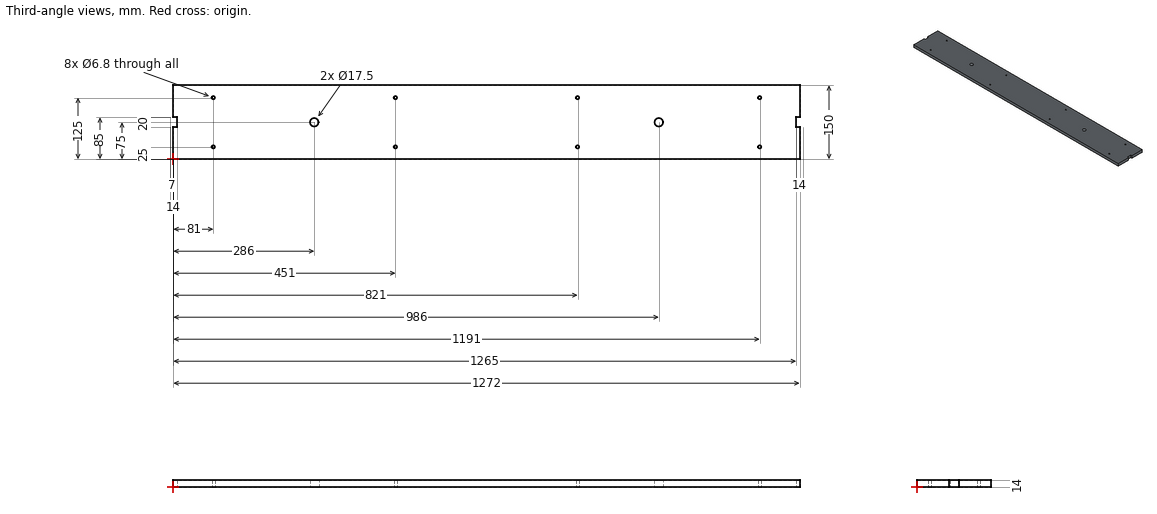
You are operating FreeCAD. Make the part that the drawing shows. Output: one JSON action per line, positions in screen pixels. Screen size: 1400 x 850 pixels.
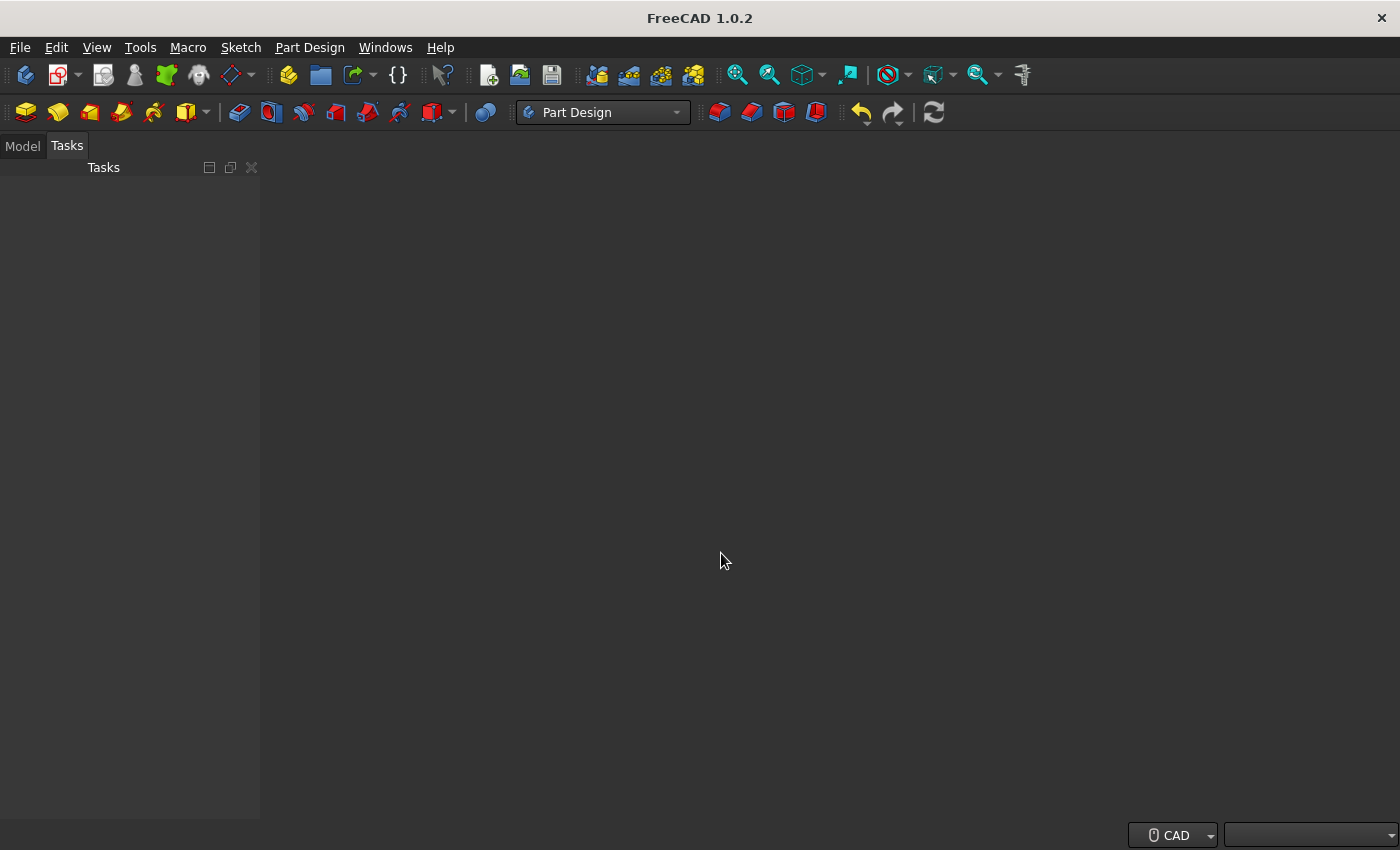
{"action": "left_click", "coordinate": [488, 76]}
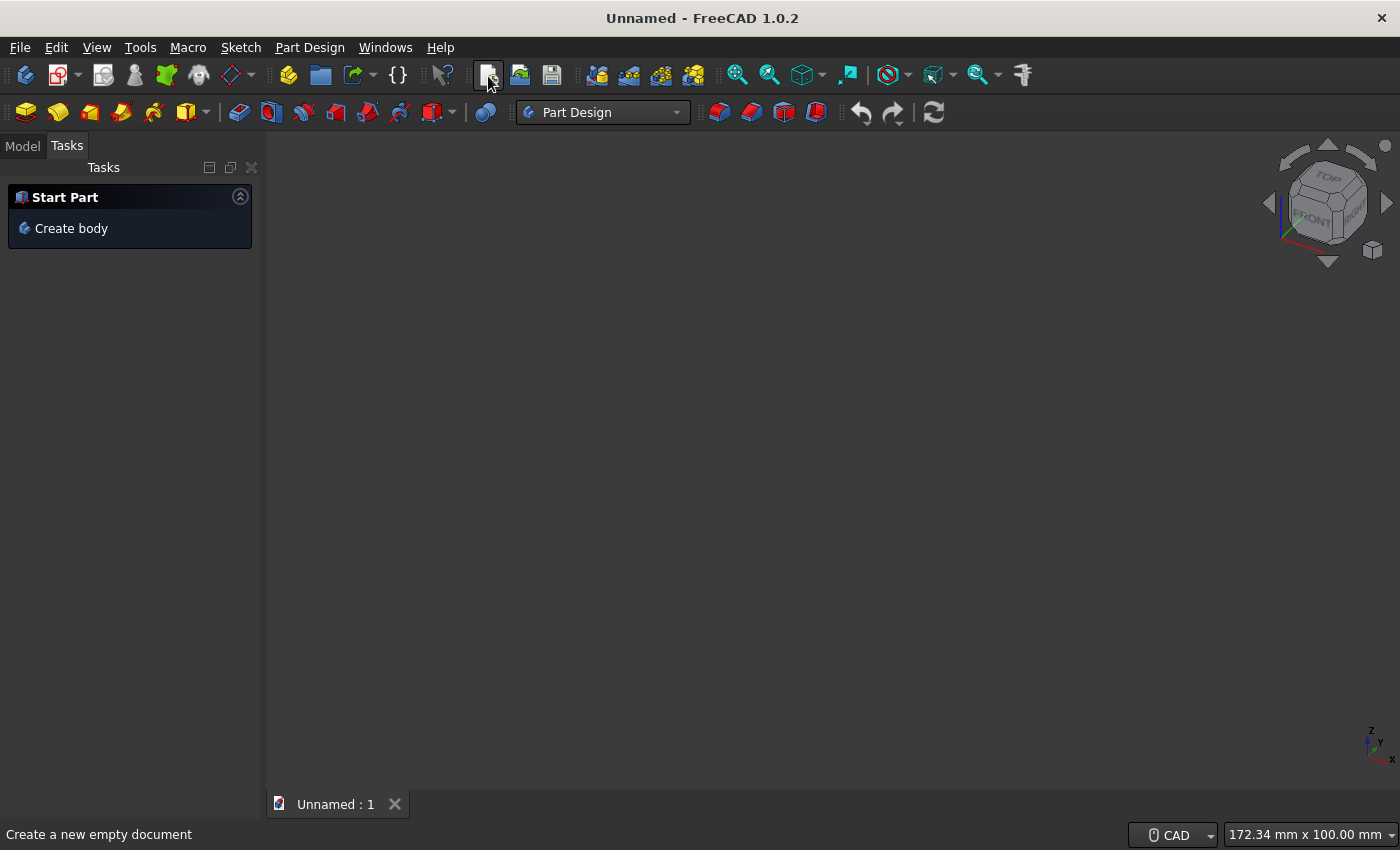
{"action": "left_click", "coordinate": [58, 76]}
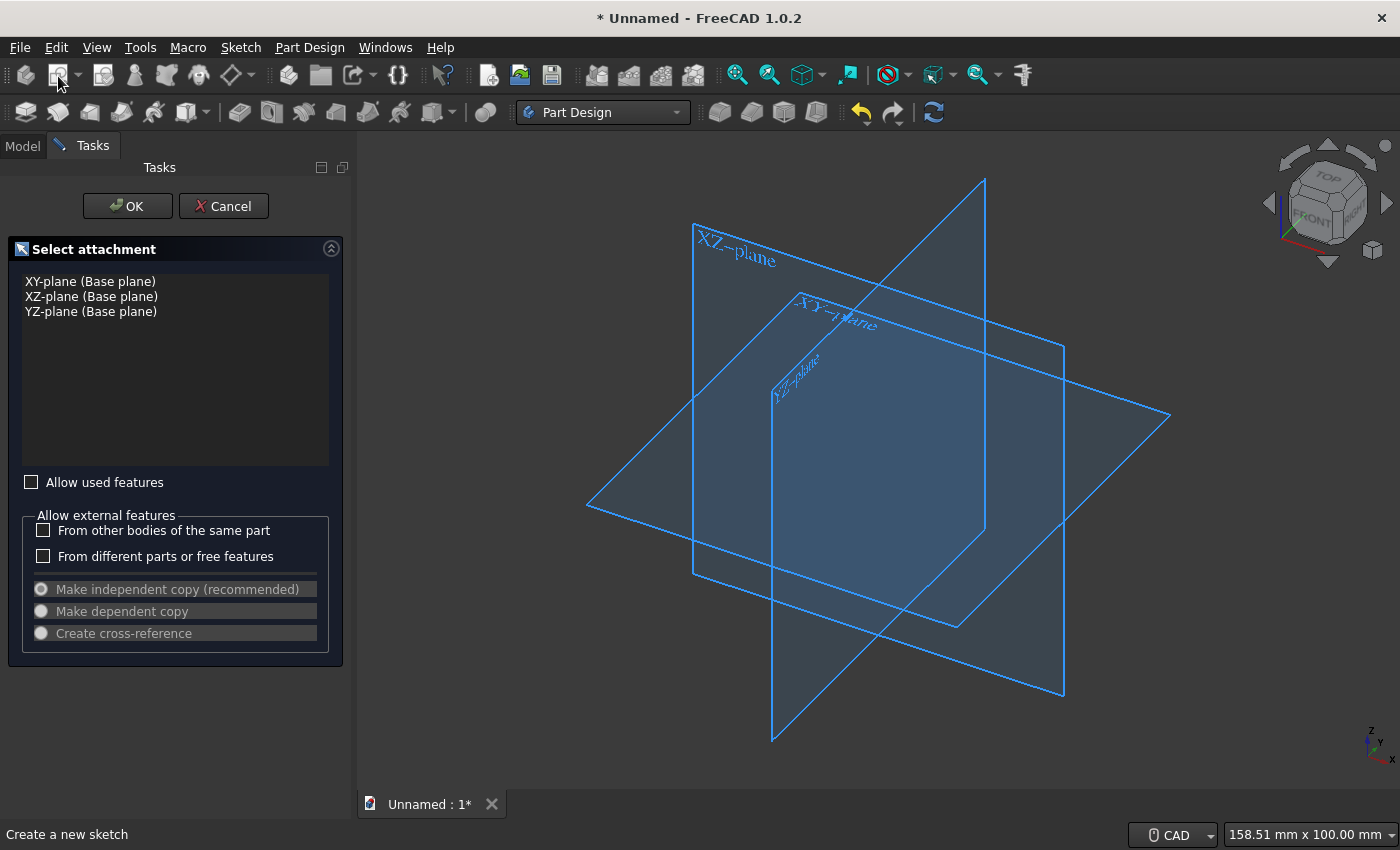
{"action": "left_click", "coordinate": [82, 282]}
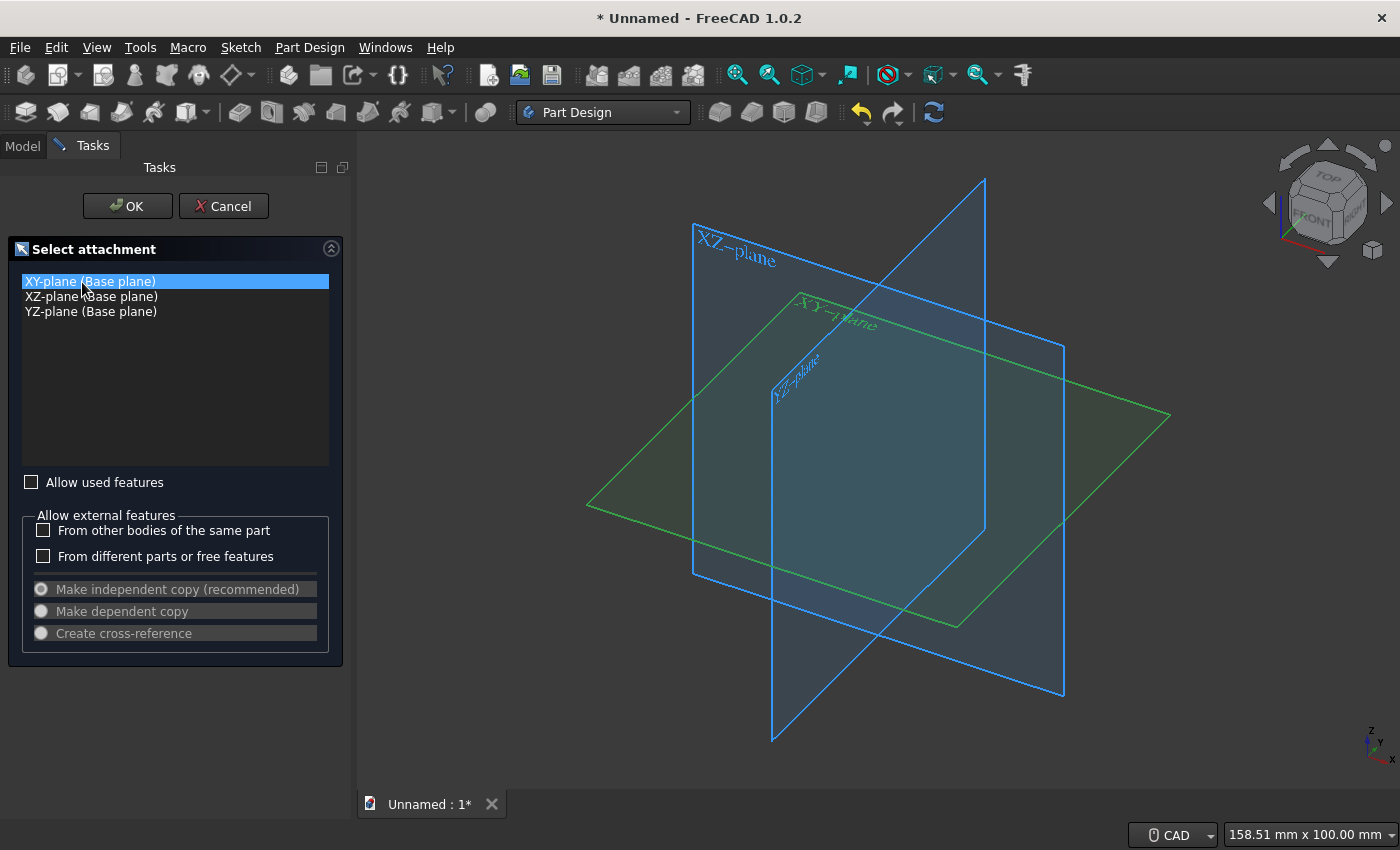
{"action": "left_click", "coordinate": [128, 206]}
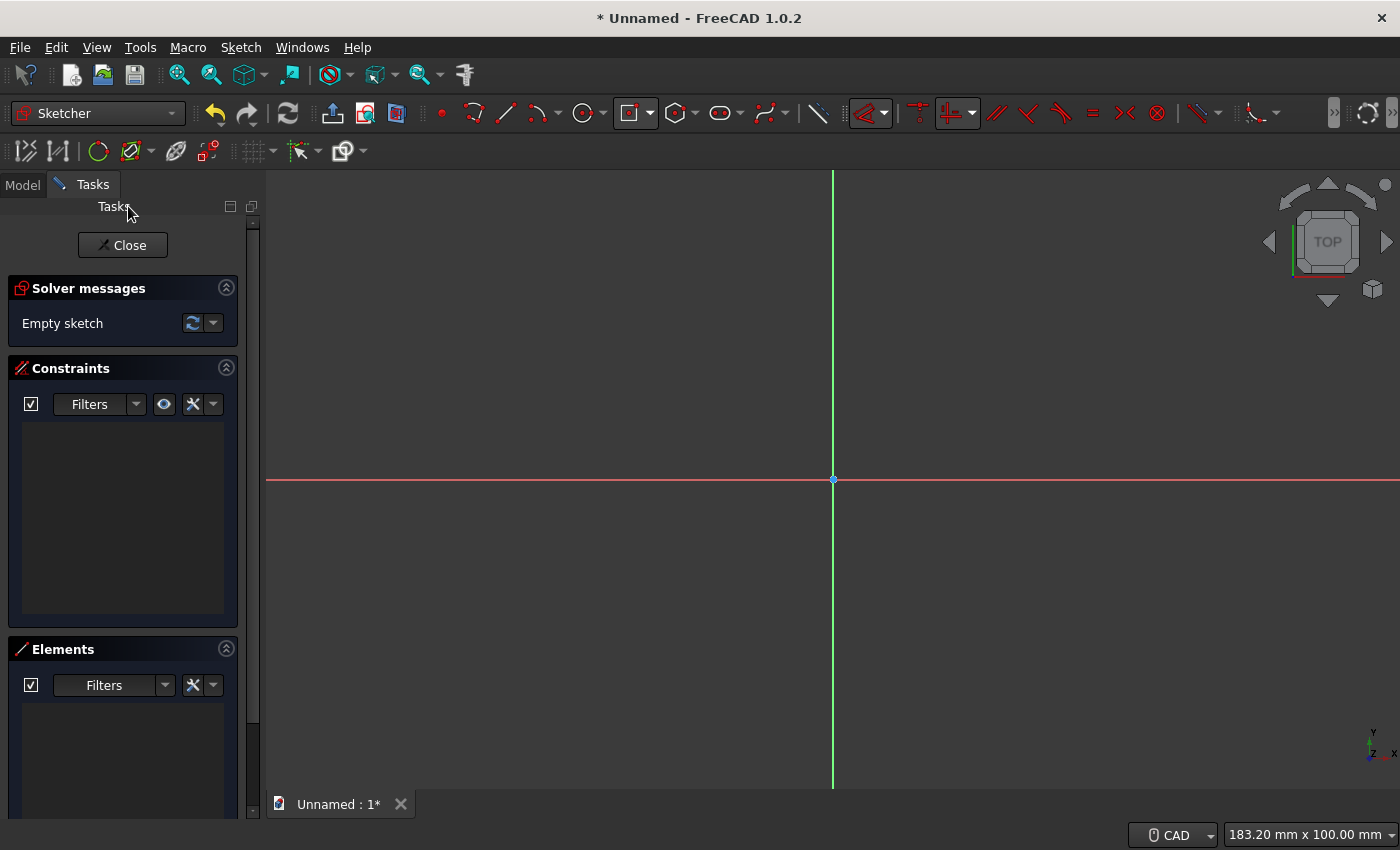
{"action": "scroll", "coordinate": [365, 526], "scroll_direction": "down", "scroll_amount": 12}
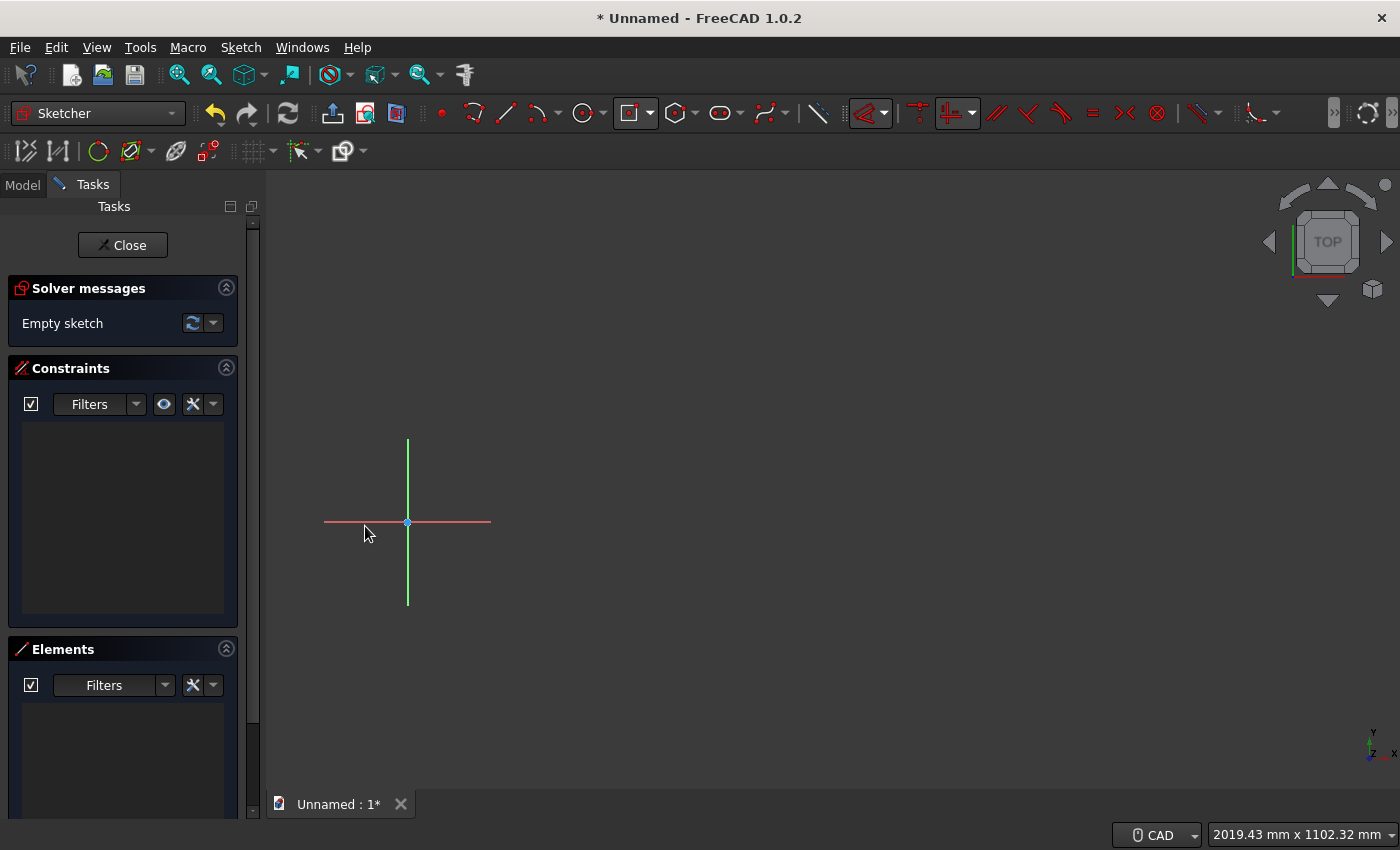
{"action": "left_click", "coordinate": [652, 114]}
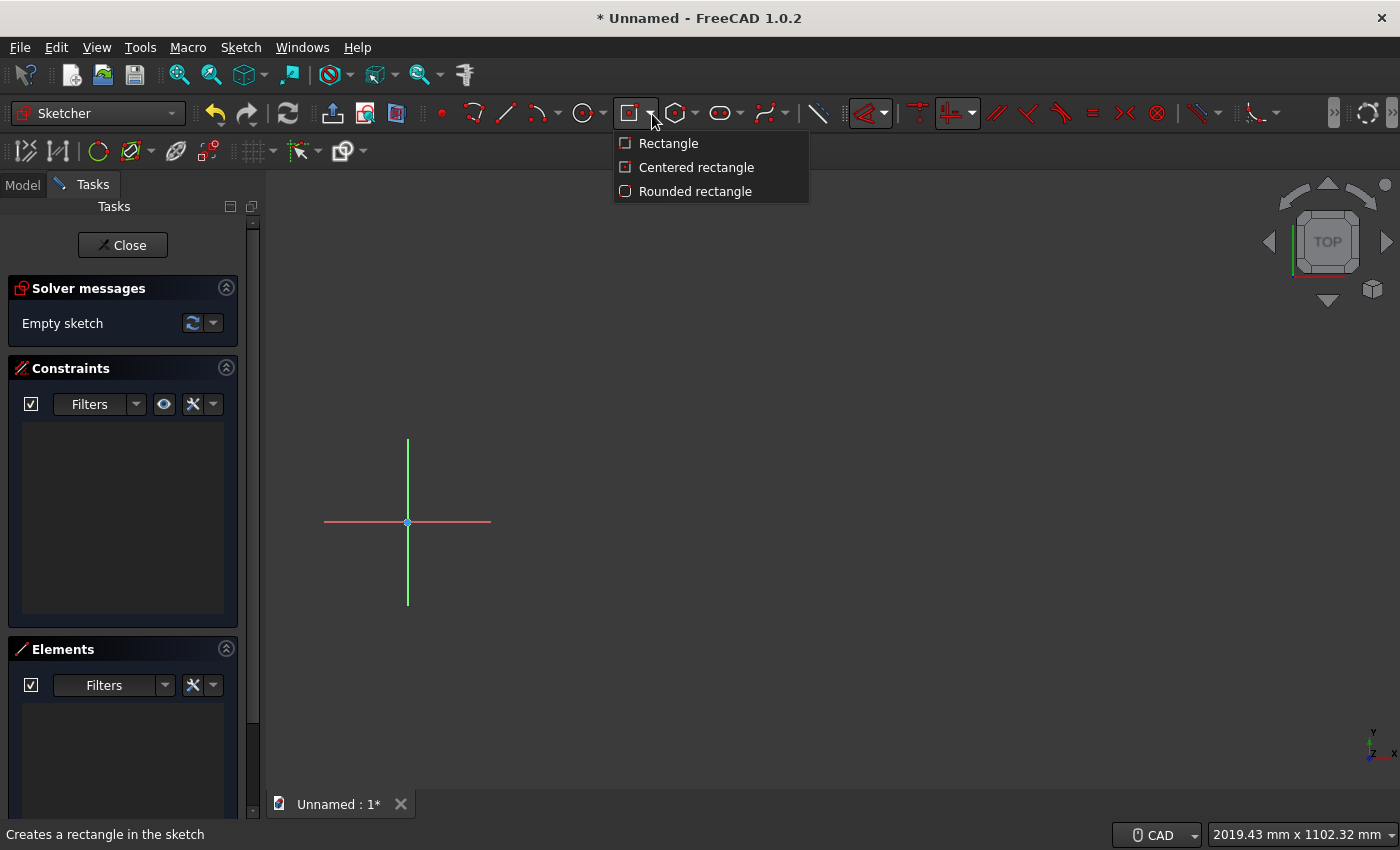
{"action": "left_click", "coordinate": [712, 143]}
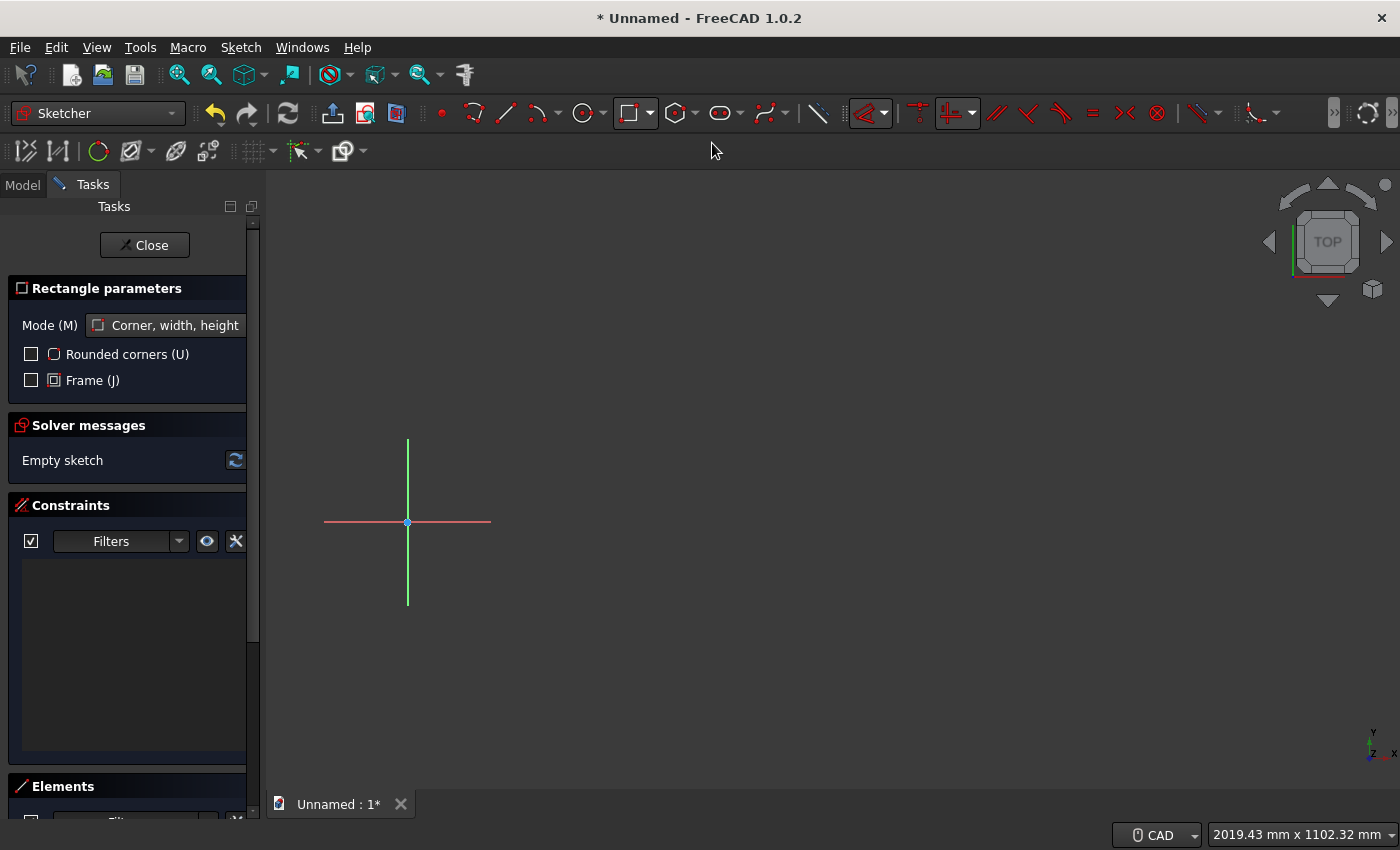
{"action": "left_click", "coordinate": [408, 522]}
{"action": "left_click", "coordinate": [1122, 438]}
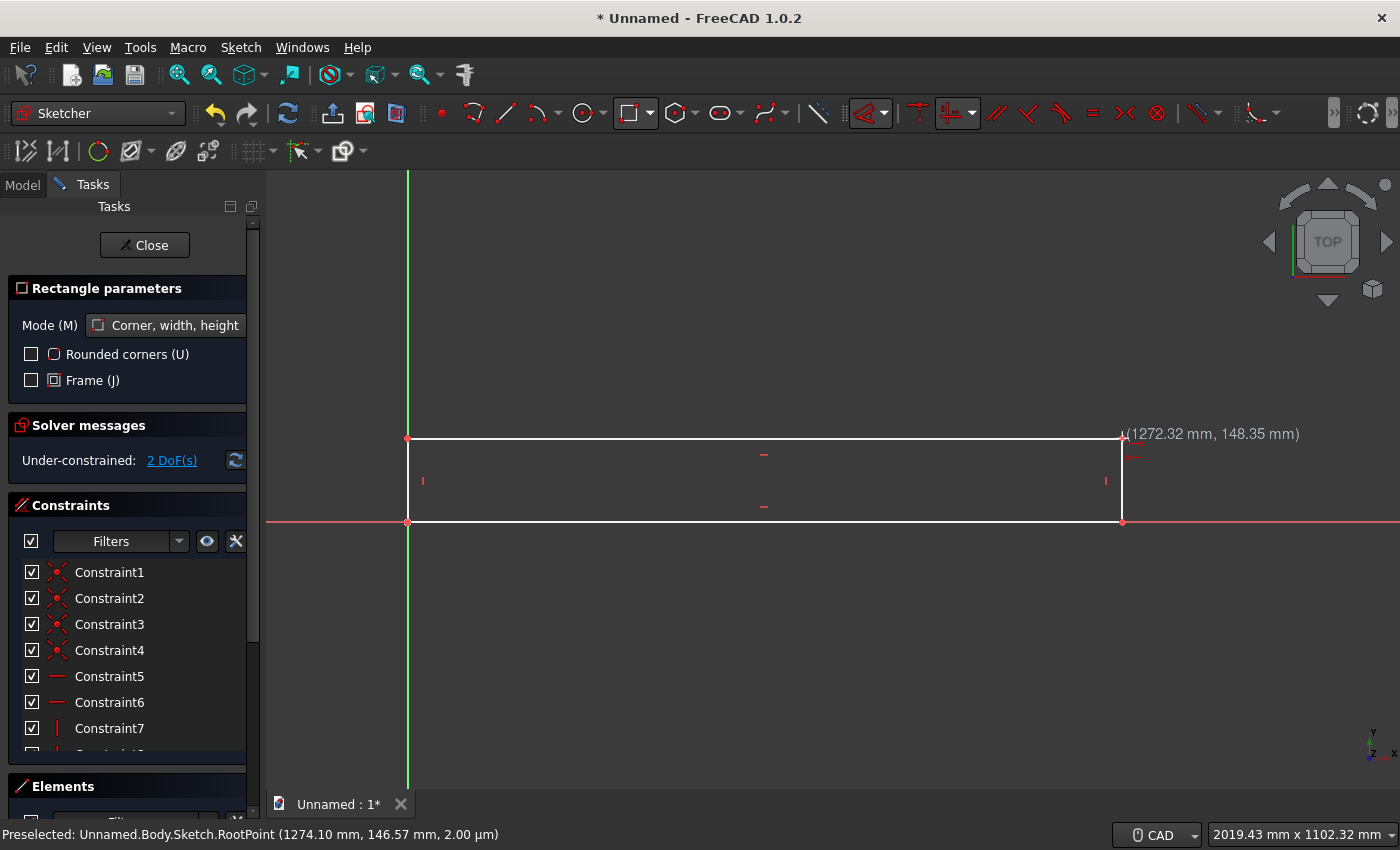
{"action": "left_click", "coordinate": [584, 114]}